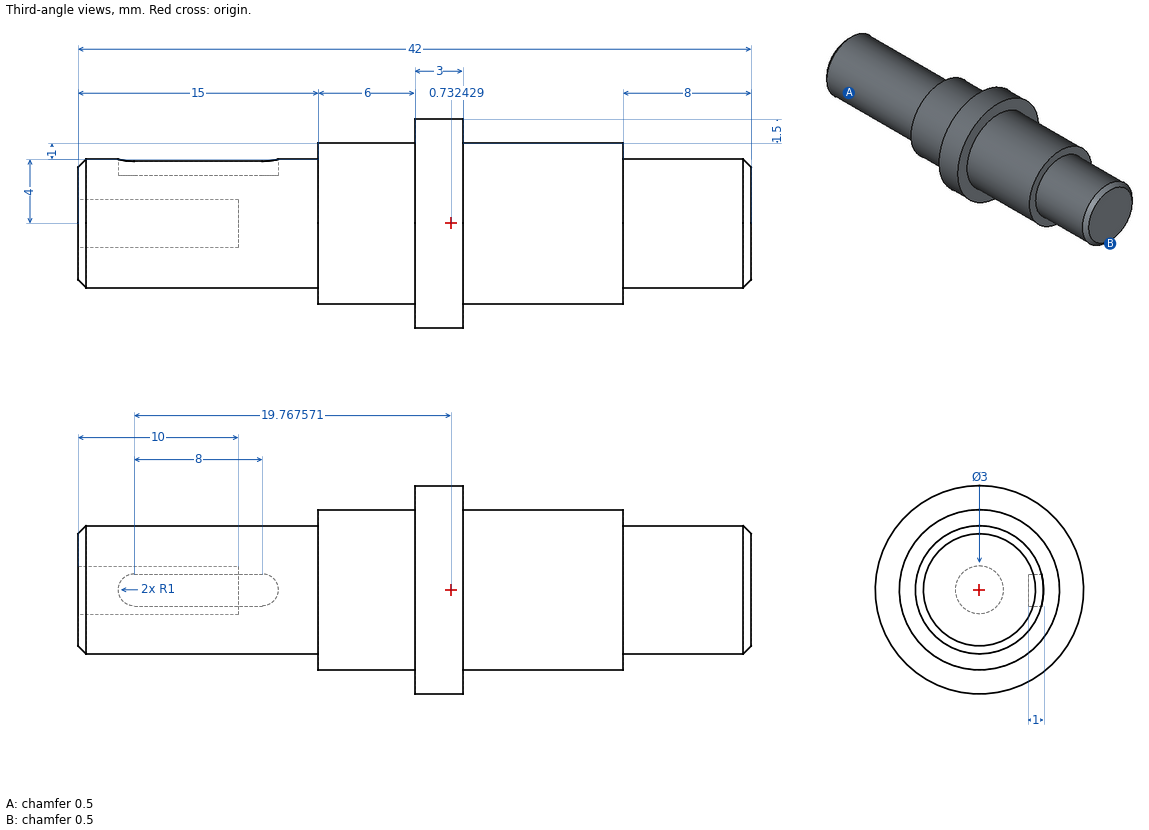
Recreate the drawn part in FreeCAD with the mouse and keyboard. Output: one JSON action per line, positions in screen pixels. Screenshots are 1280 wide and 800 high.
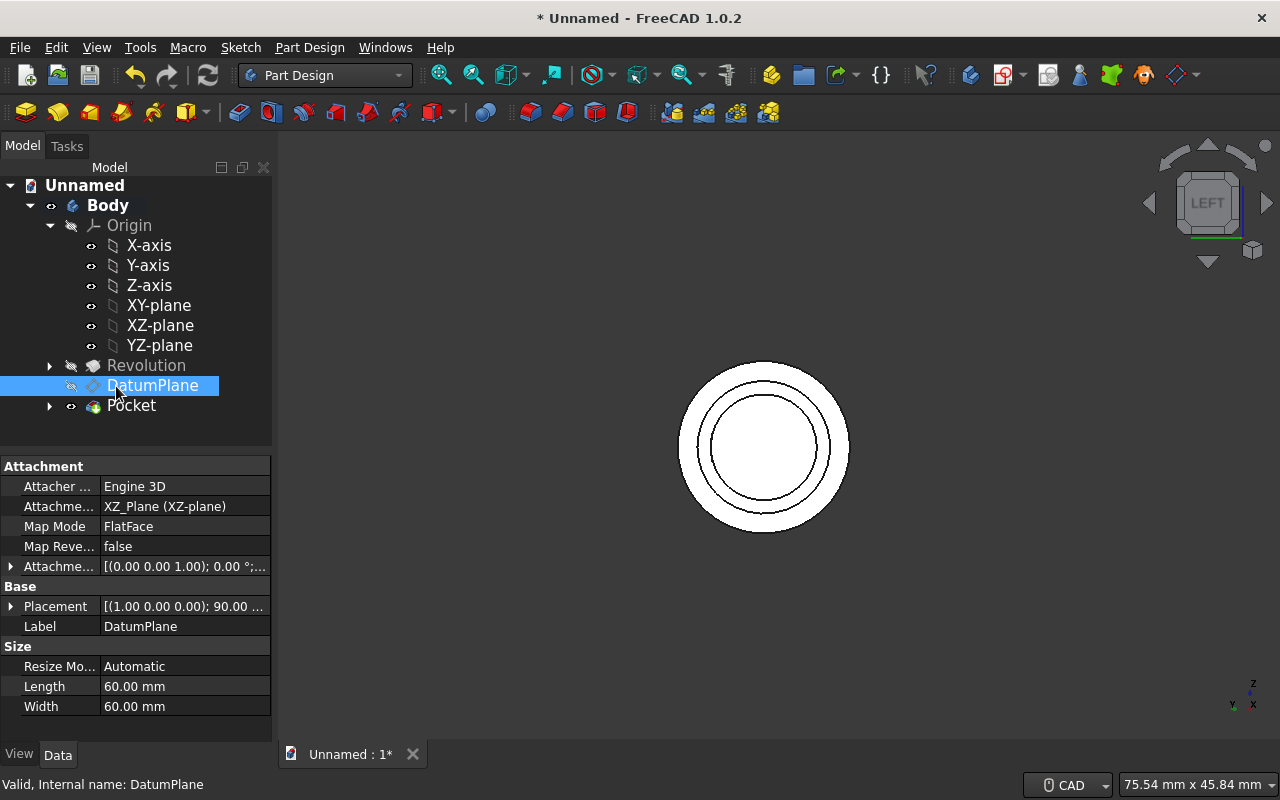
{"action": "left_click", "coordinate": [442, 76]}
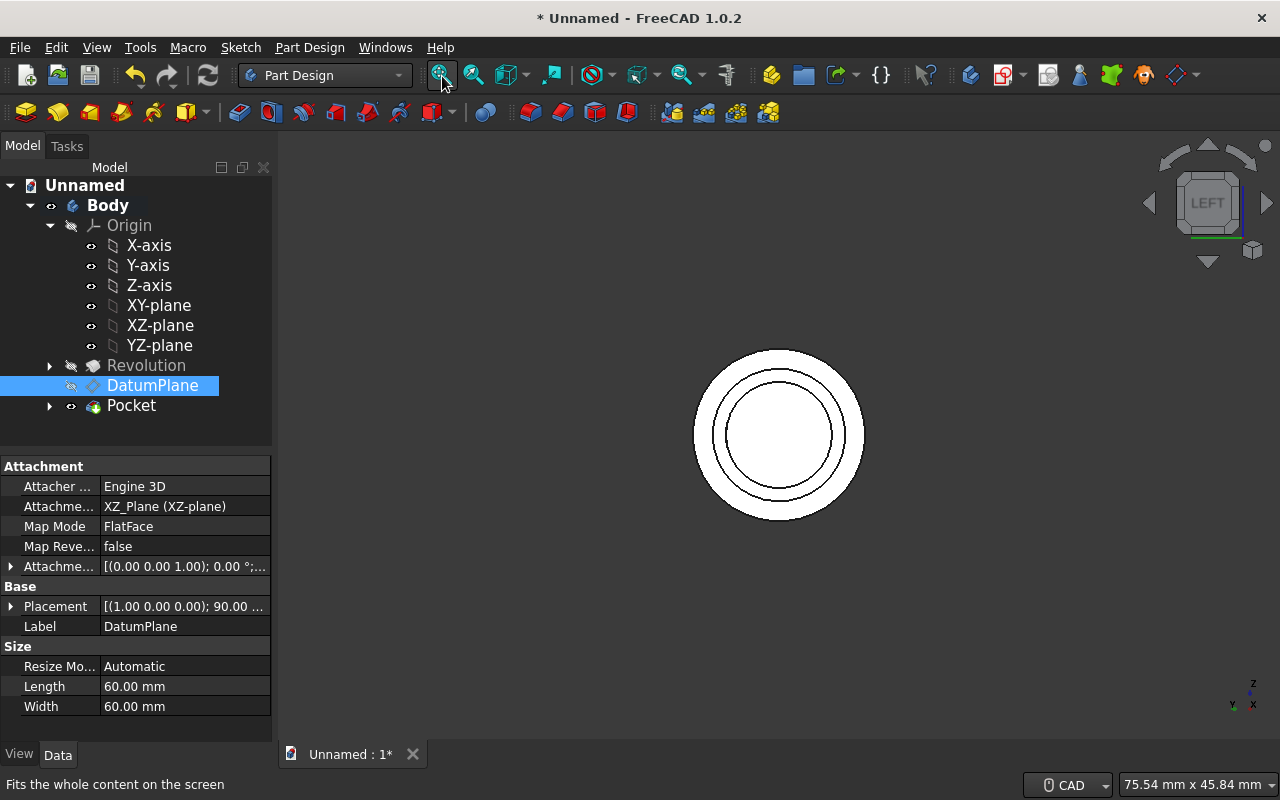
{"action": "left_click", "coordinate": [779, 434]}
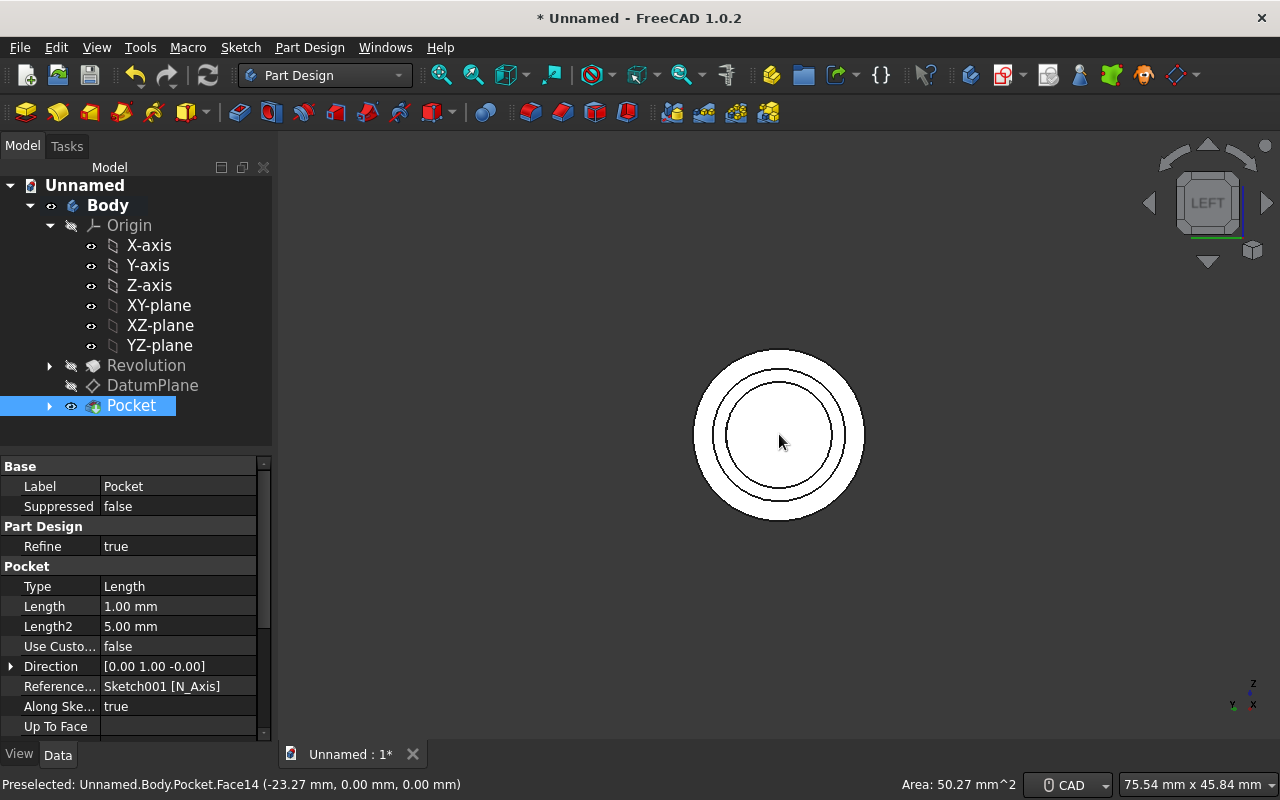
{"action": "left_click", "coordinate": [1004, 76]}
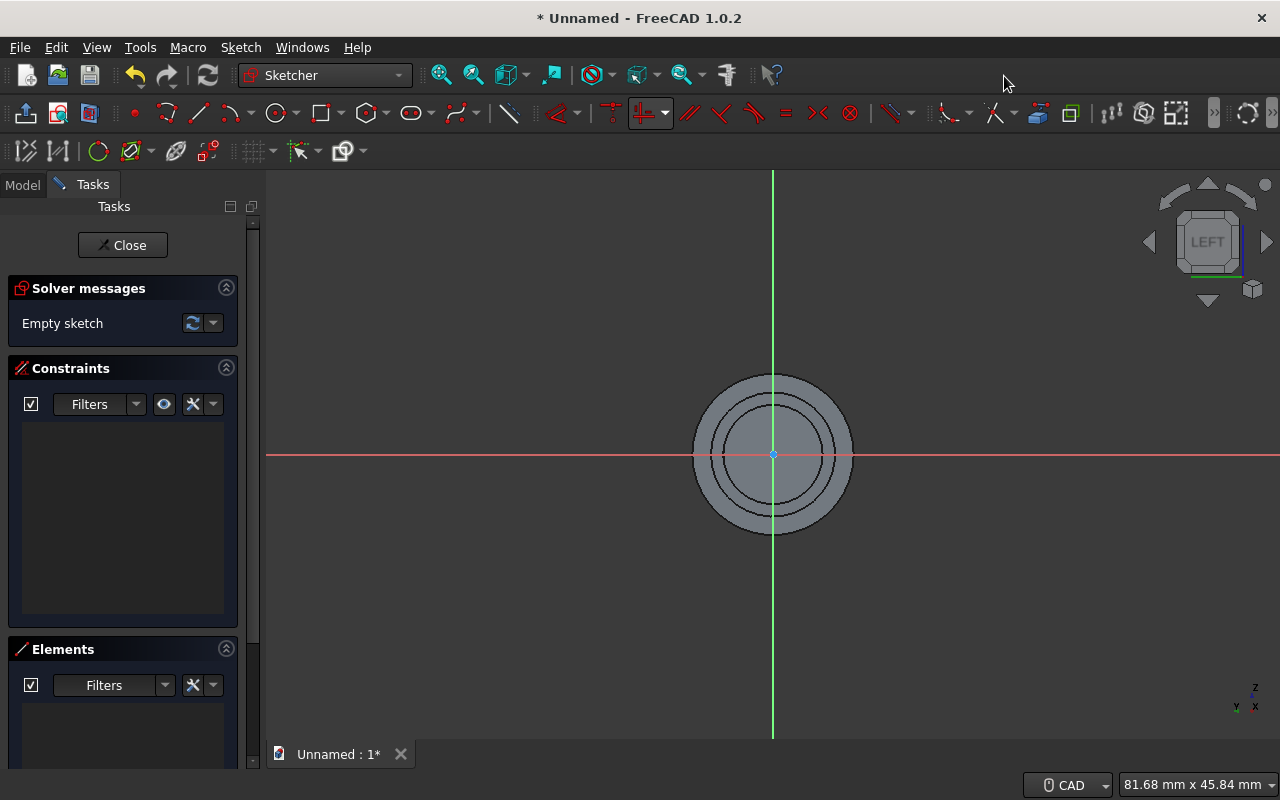
{"action": "scroll", "coordinate": [782, 454], "scroll_direction": "up", "scroll_amount": 11}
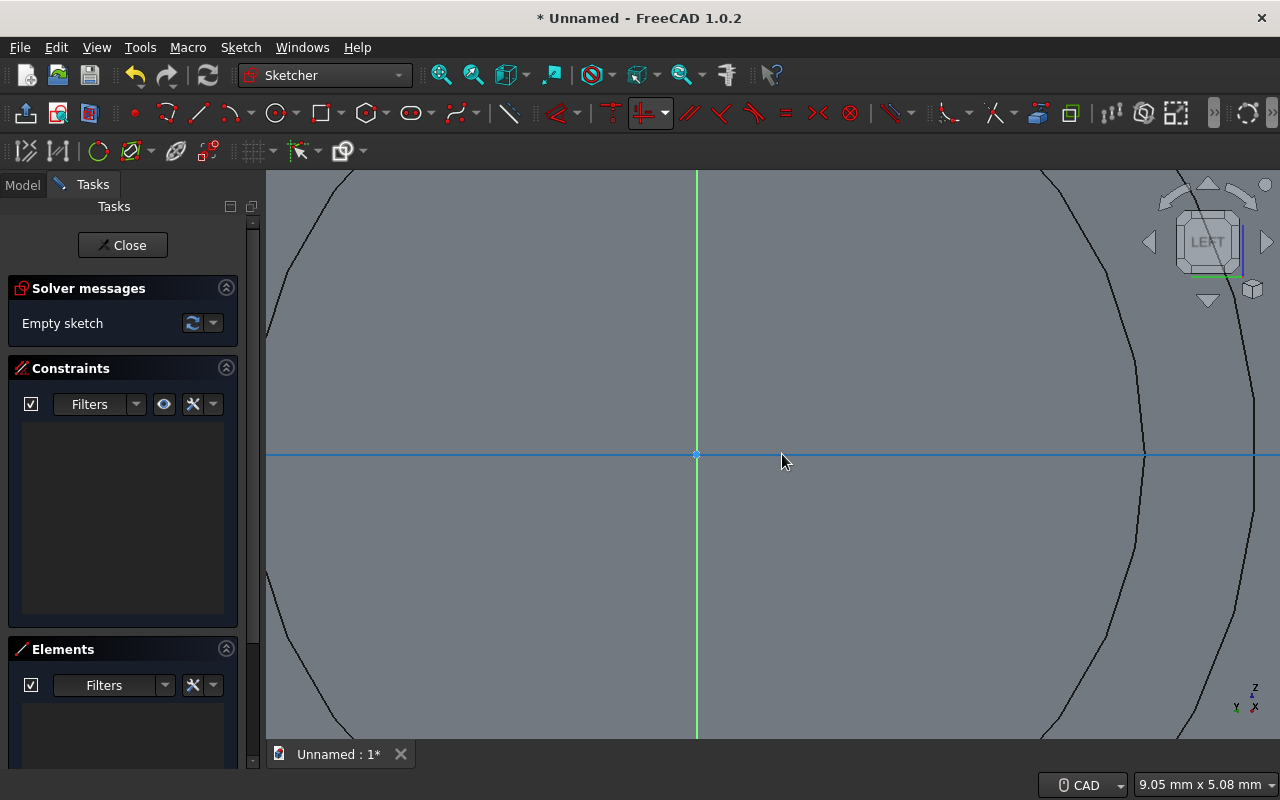
{"action": "left_click", "coordinate": [276, 114]}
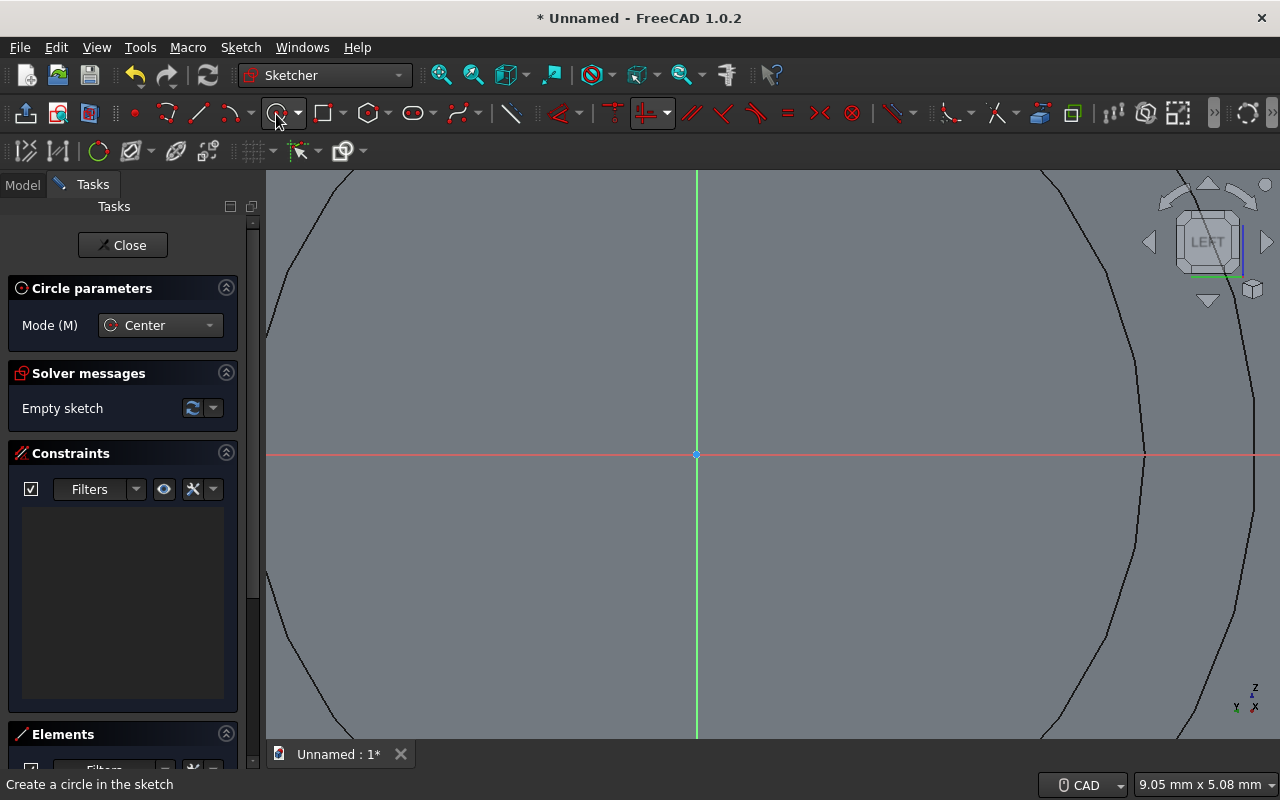
{"action": "left_click", "coordinate": [697, 454]}
{"action": "mouse_move", "coordinate": [816, 336]}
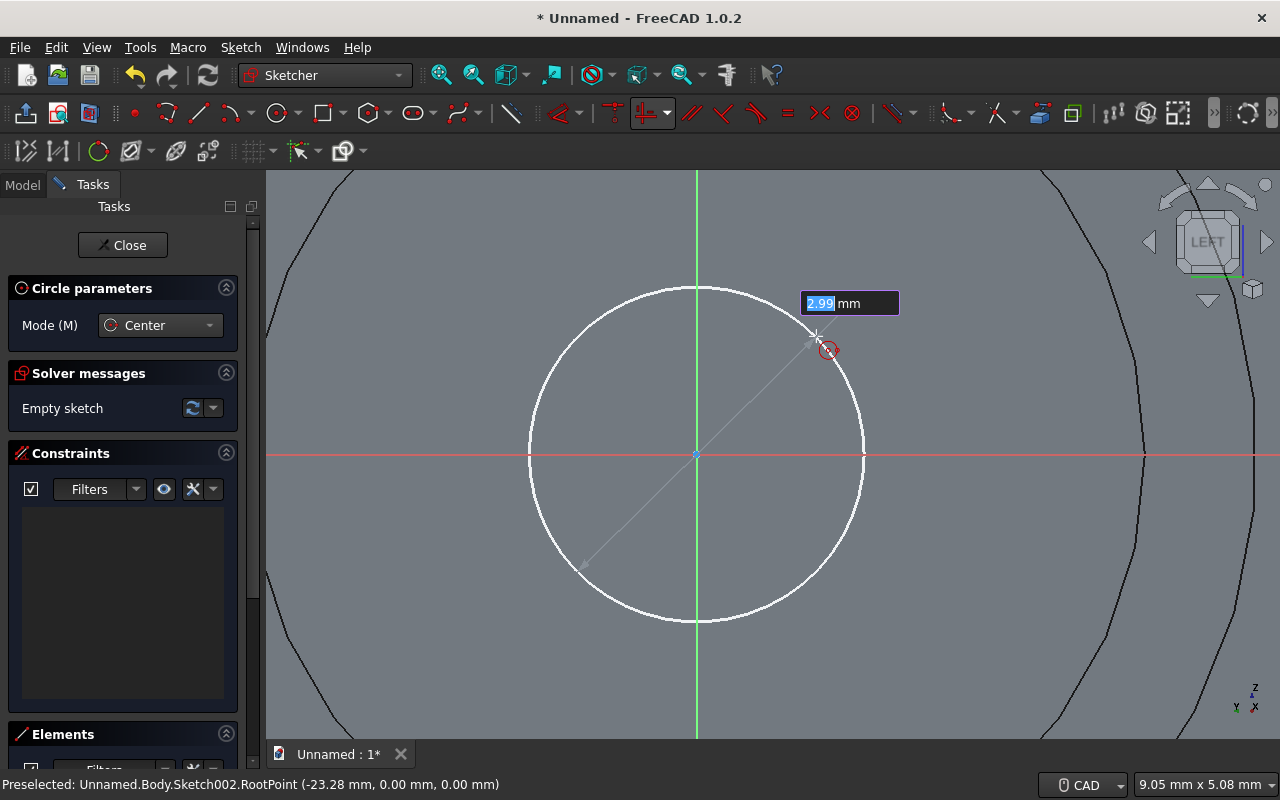
{"action": "type", "text": "3"}
{"action": "key", "text": "Return"}
{"action": "key", "text": "Escape"}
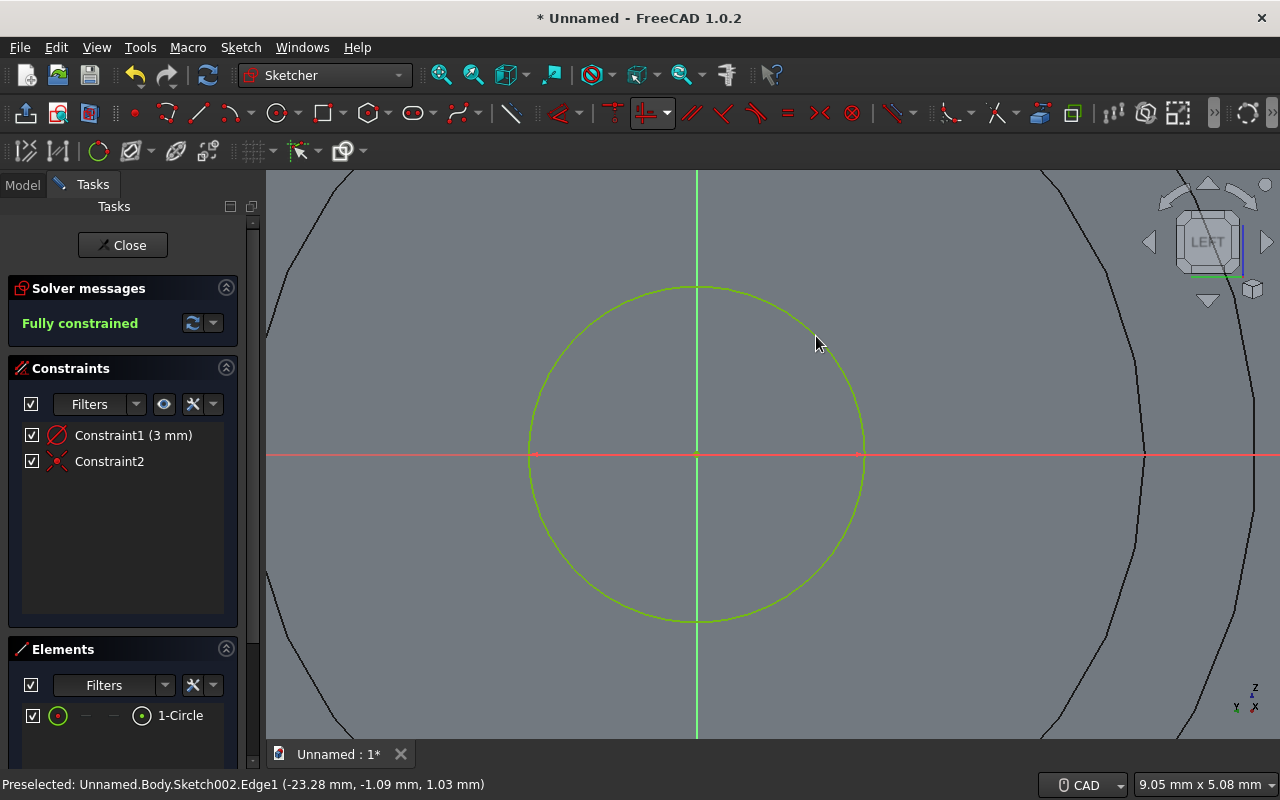
{"action": "left_click", "coordinate": [123, 245]}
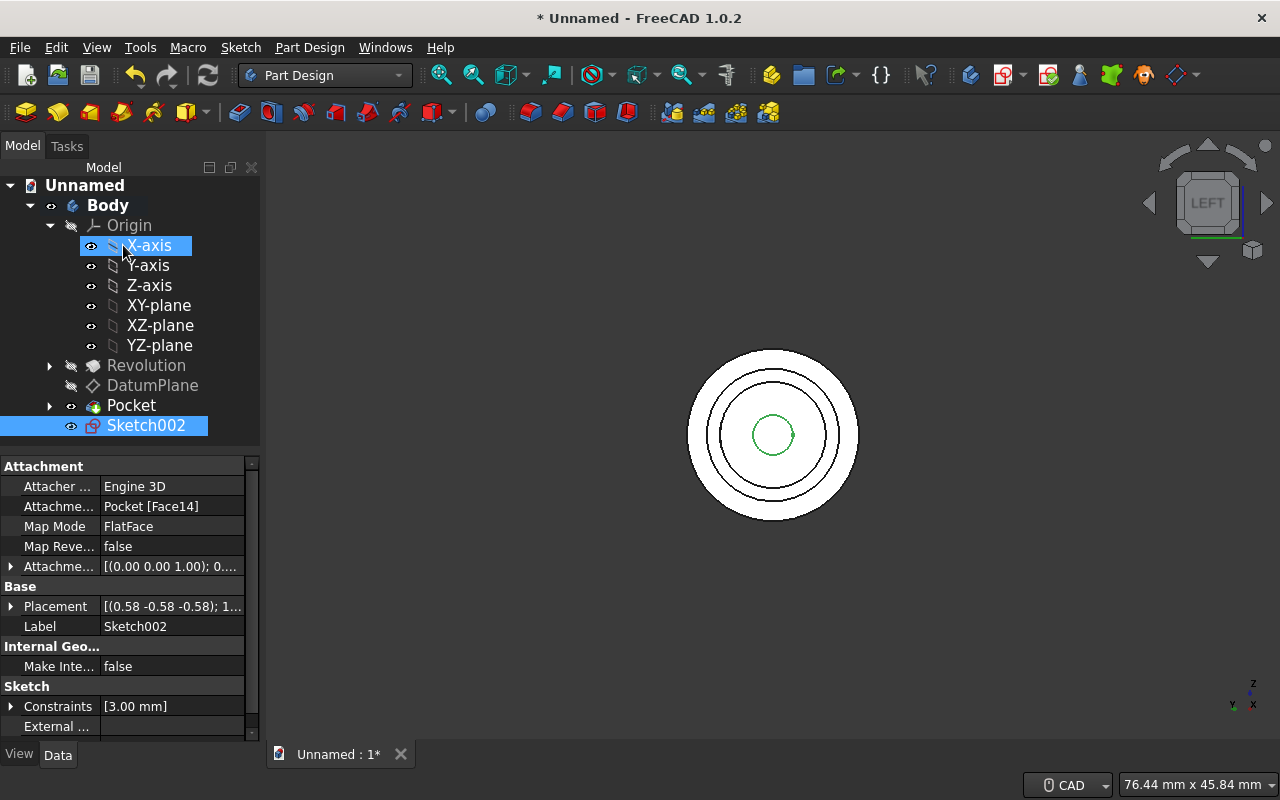
{"action": "left_click", "coordinate": [240, 112]}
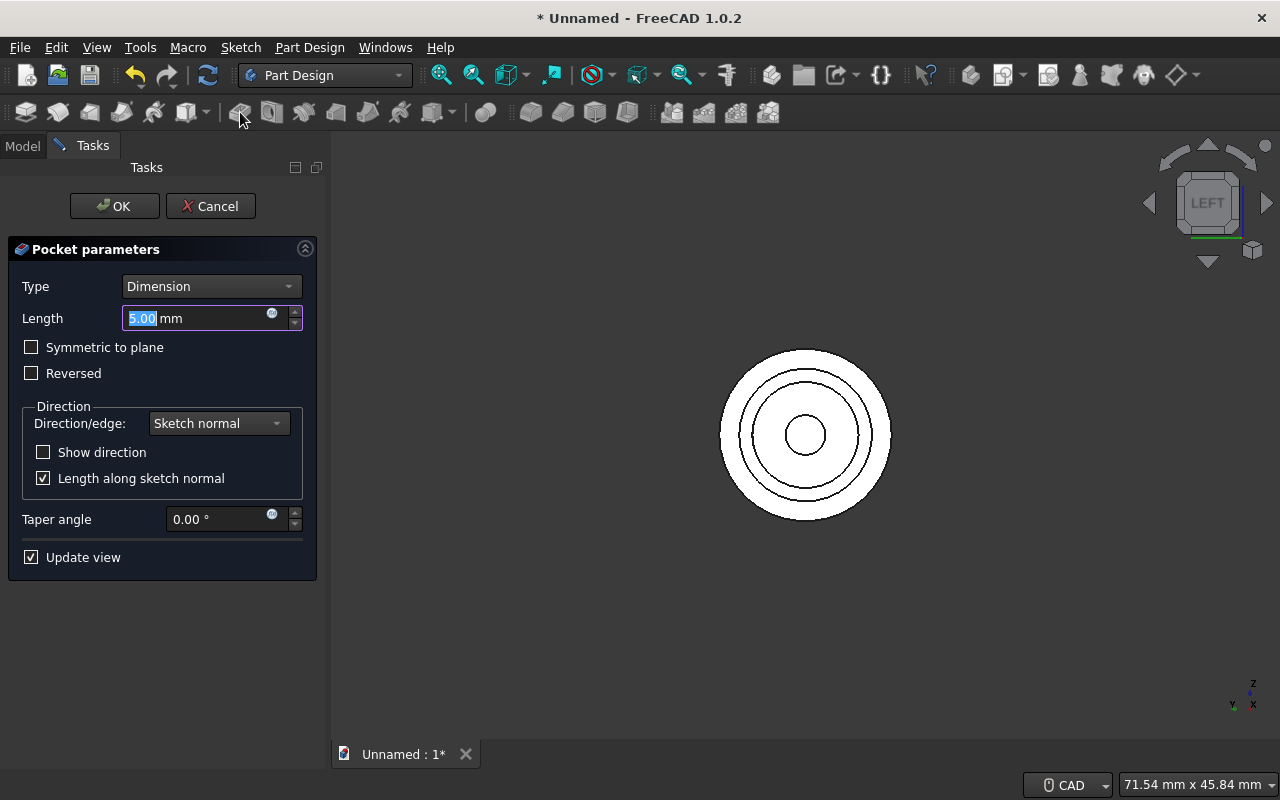
{"action": "type", "text": "10"}
{"action": "key", "text": "Tab"}